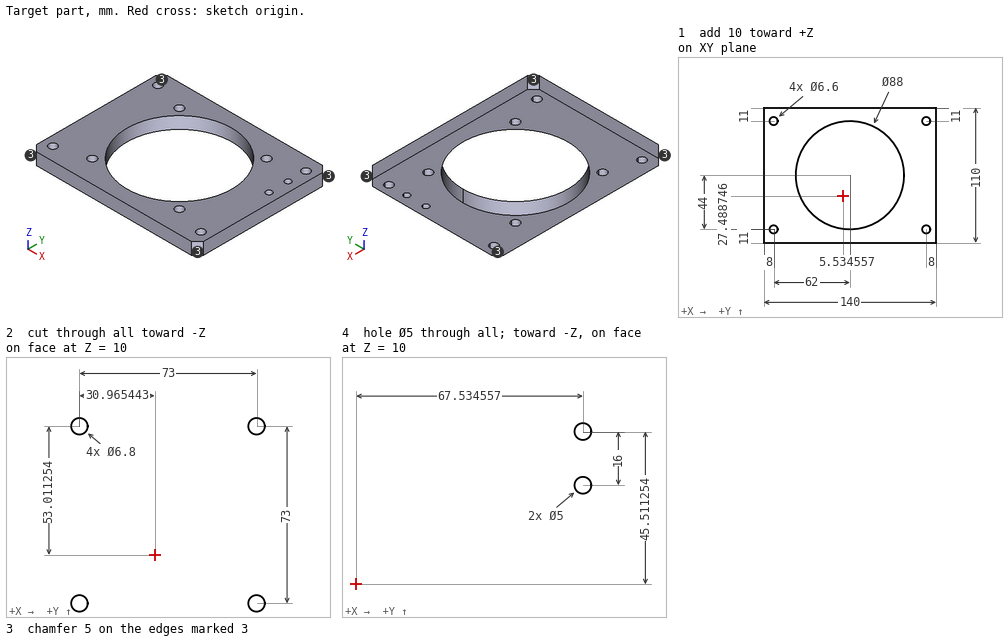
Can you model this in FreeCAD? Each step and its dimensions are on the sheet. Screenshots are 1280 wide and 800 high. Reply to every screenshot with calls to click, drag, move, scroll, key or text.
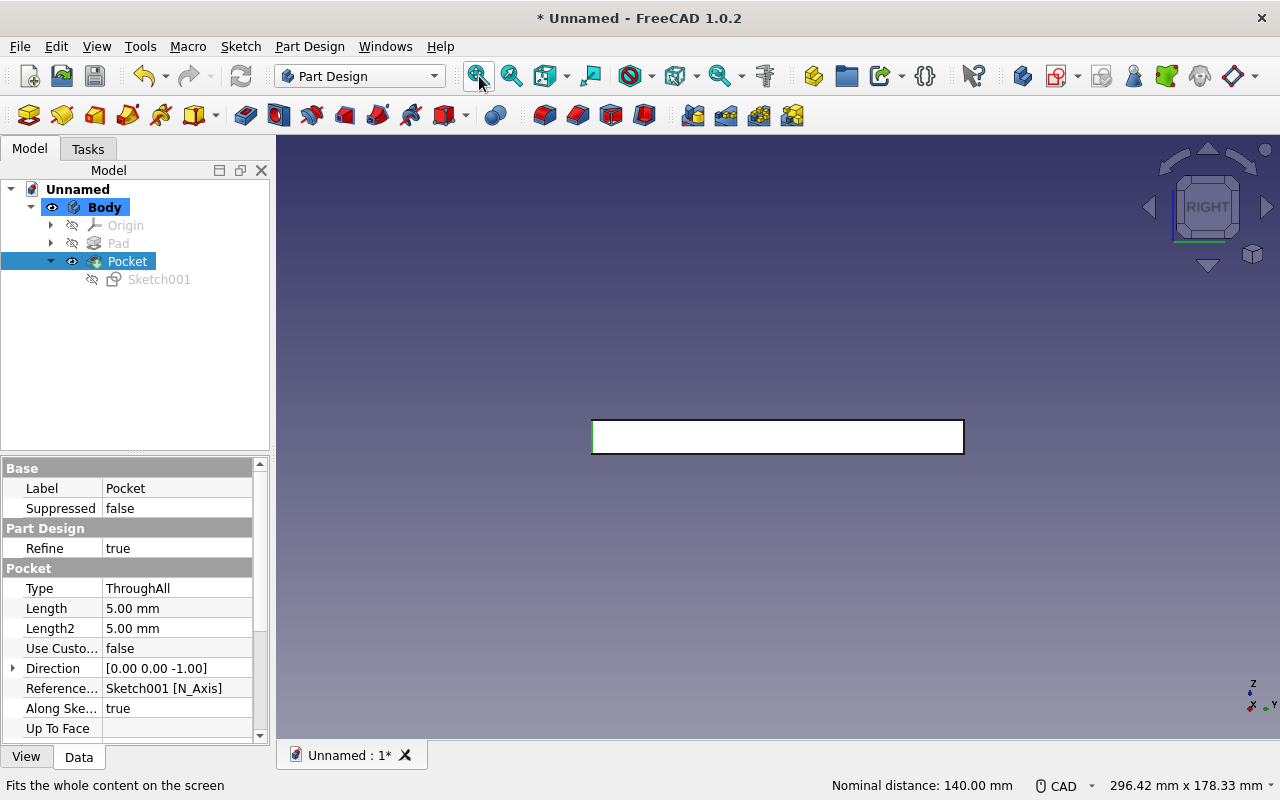
click(964, 436, ctrl)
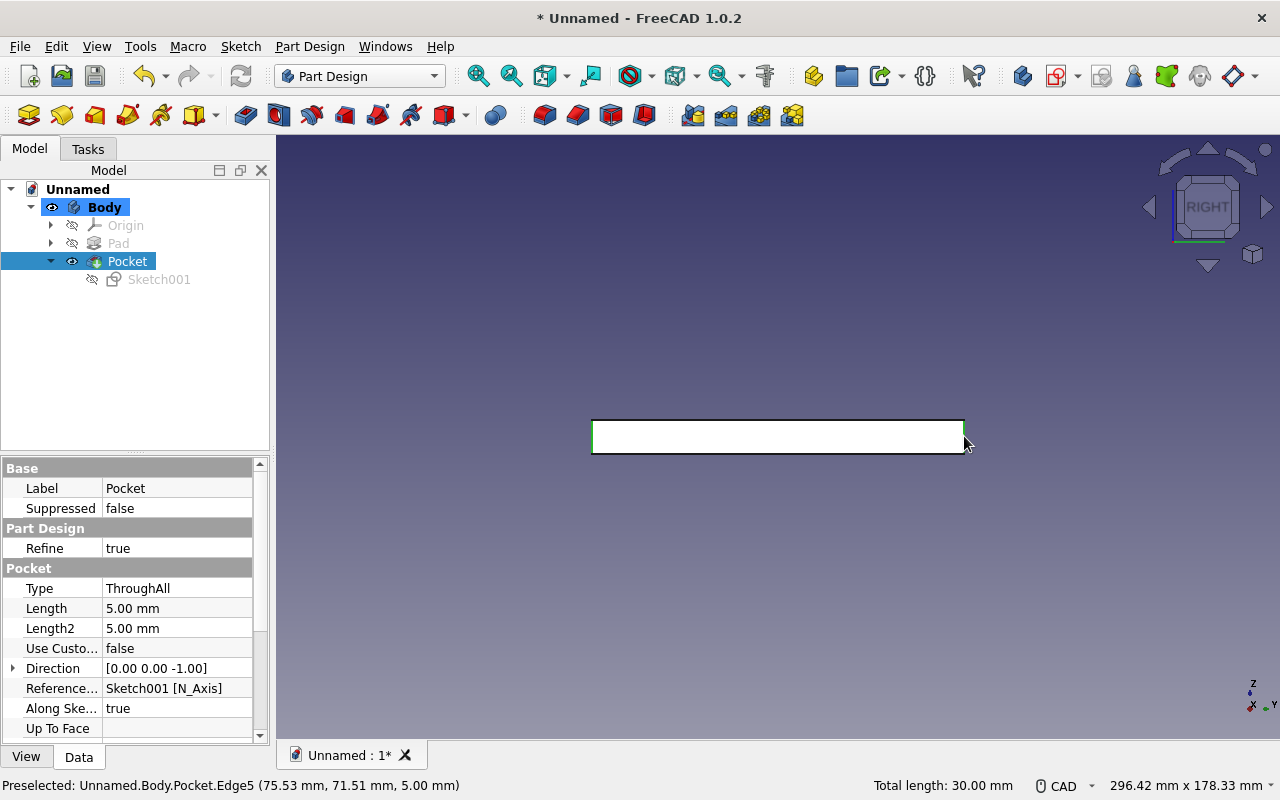
key(5)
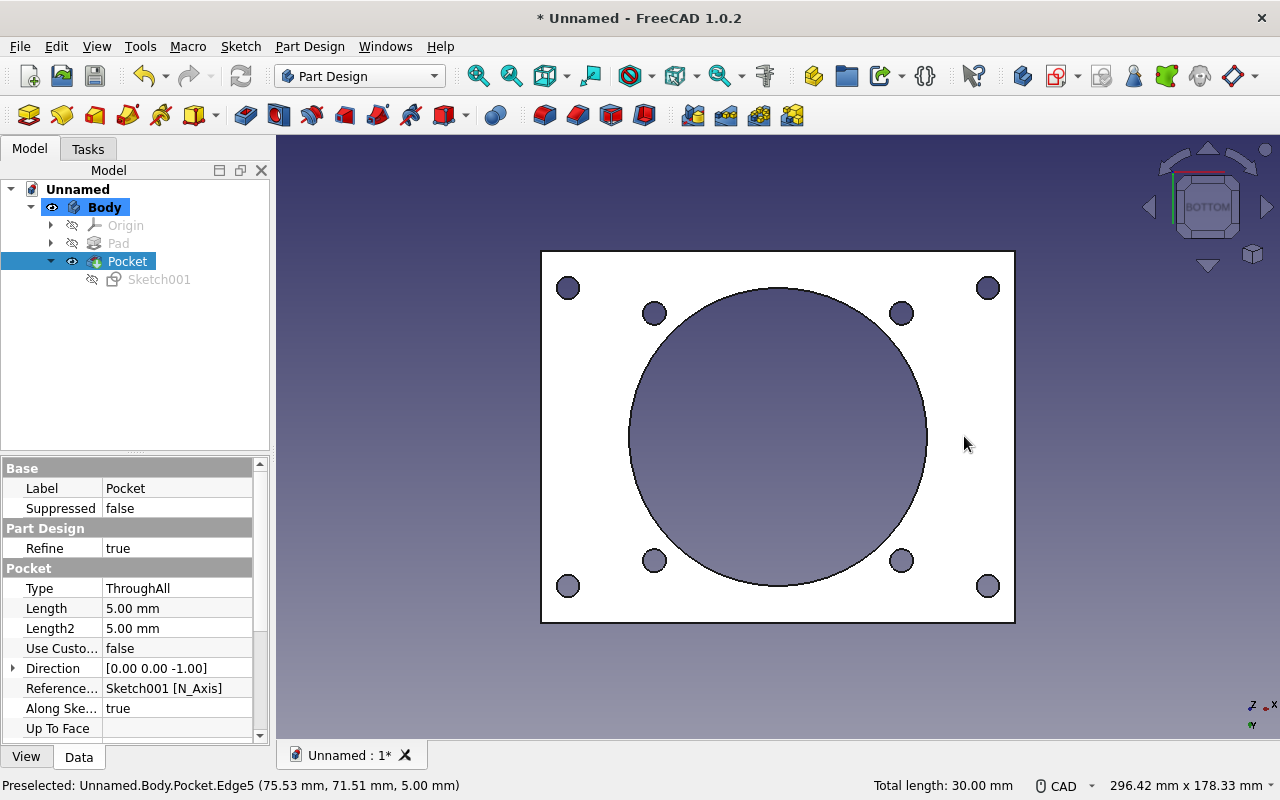
key(4)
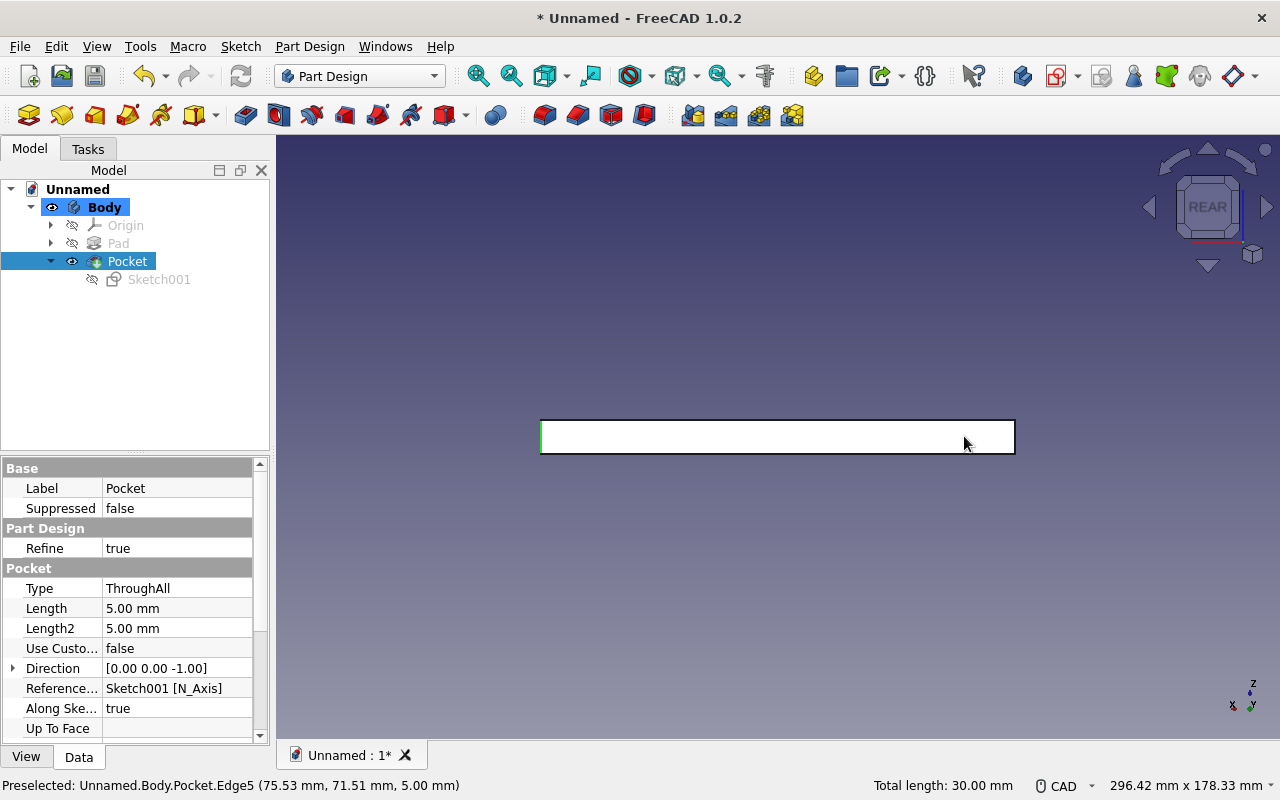
click(1015, 436, ctrl)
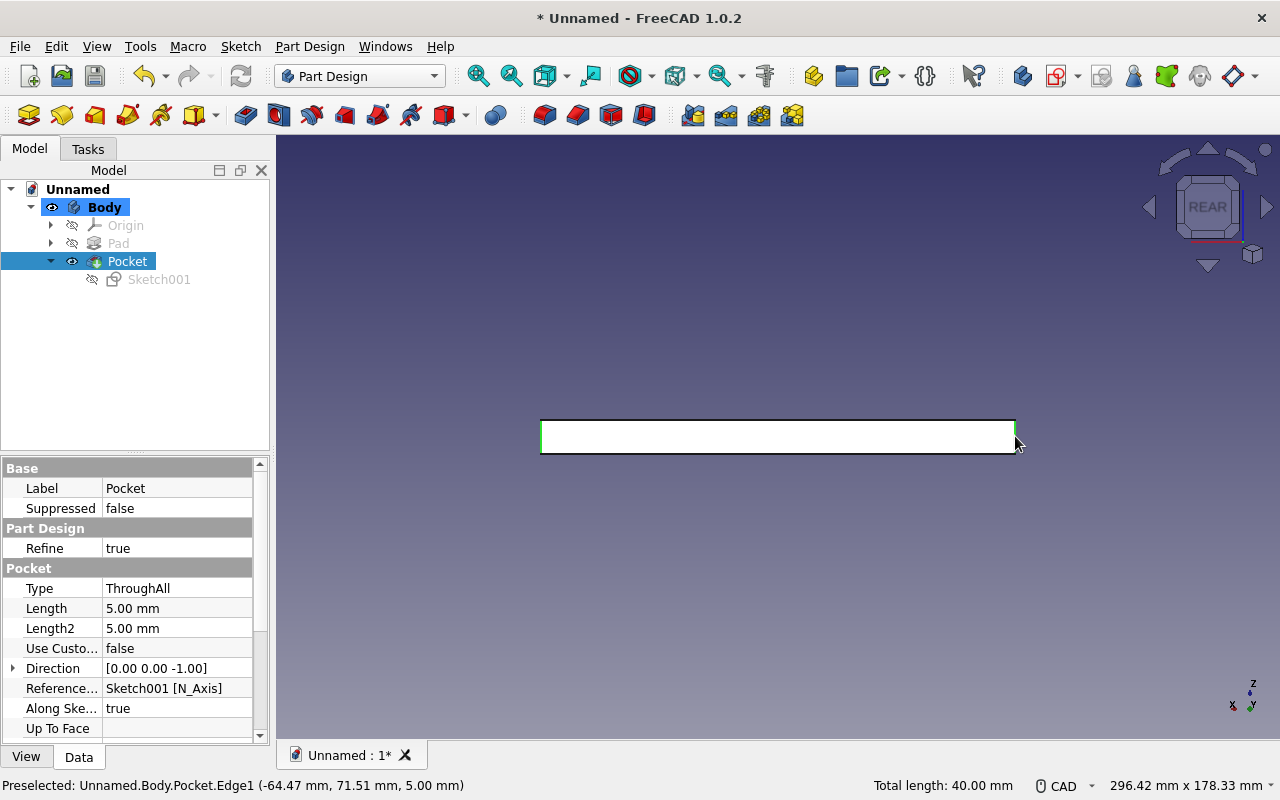
click(578, 116)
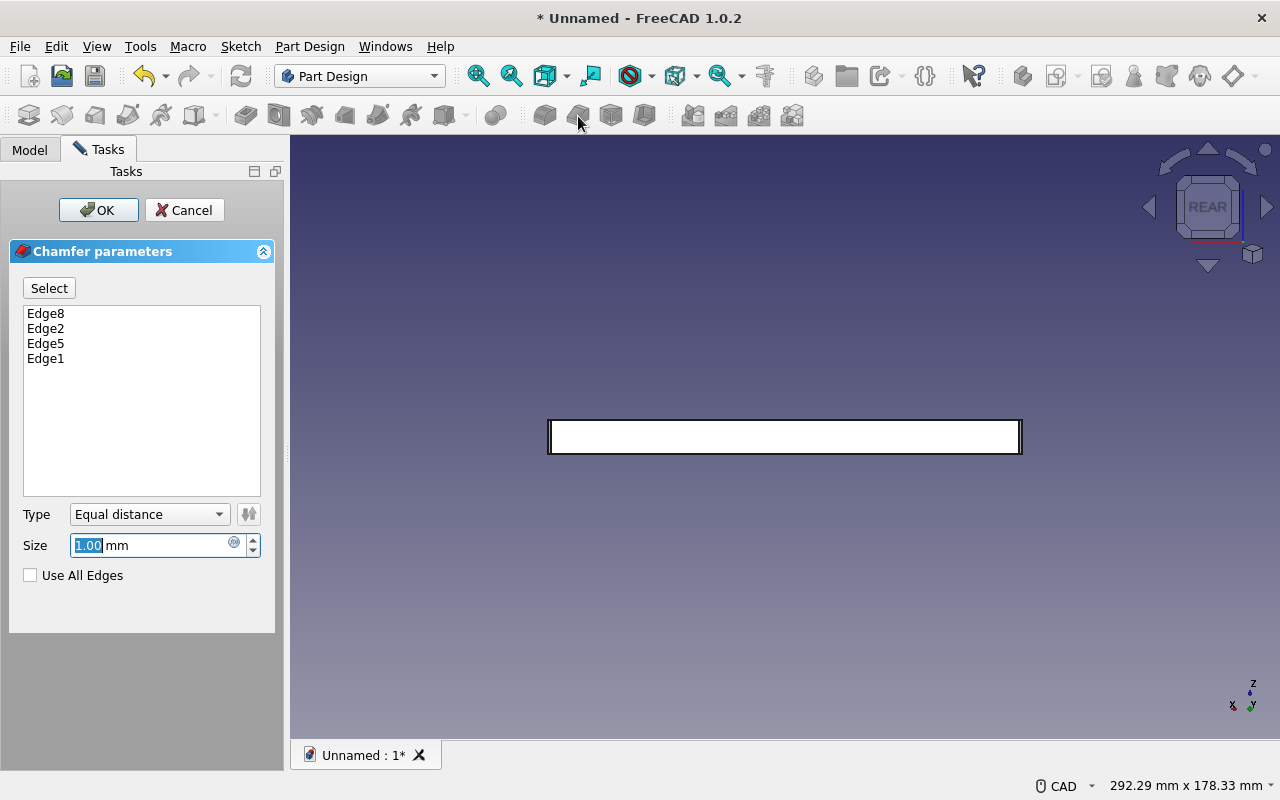
text(5)
key(Tab)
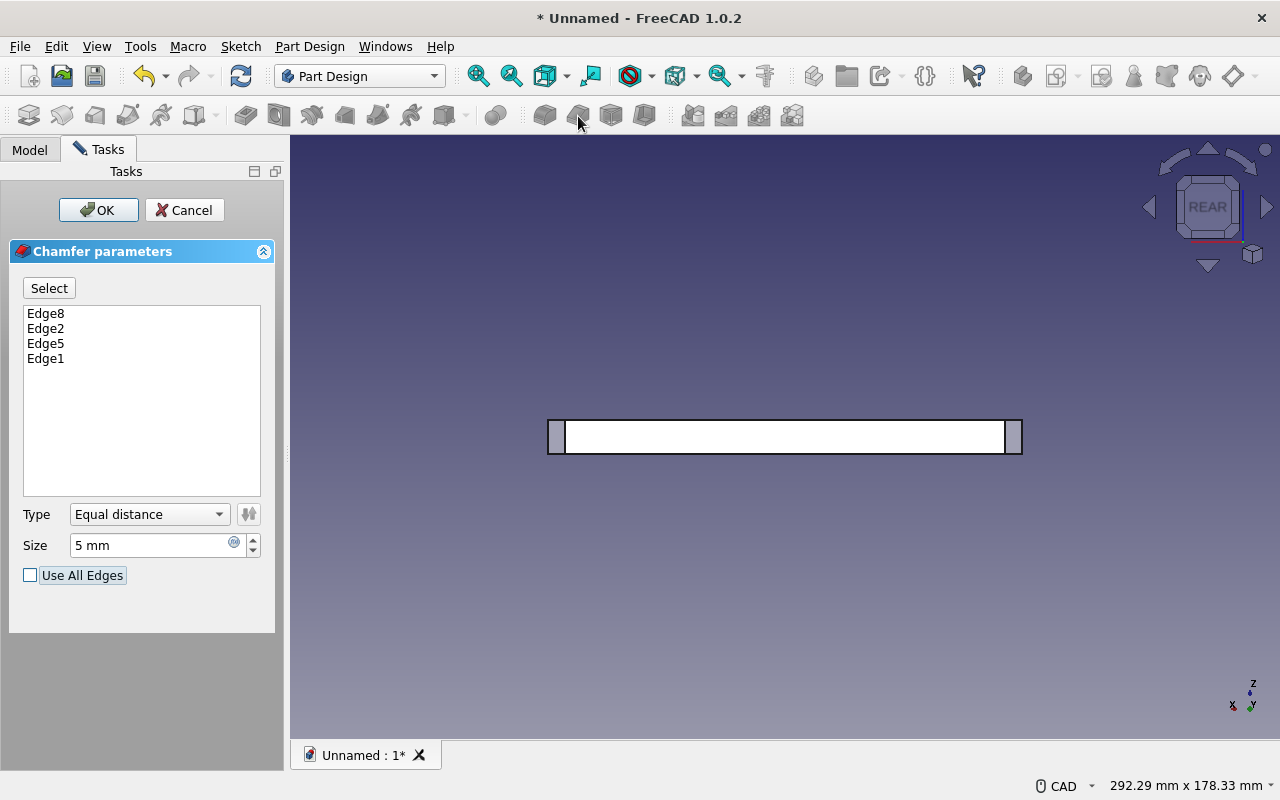
click(99, 210)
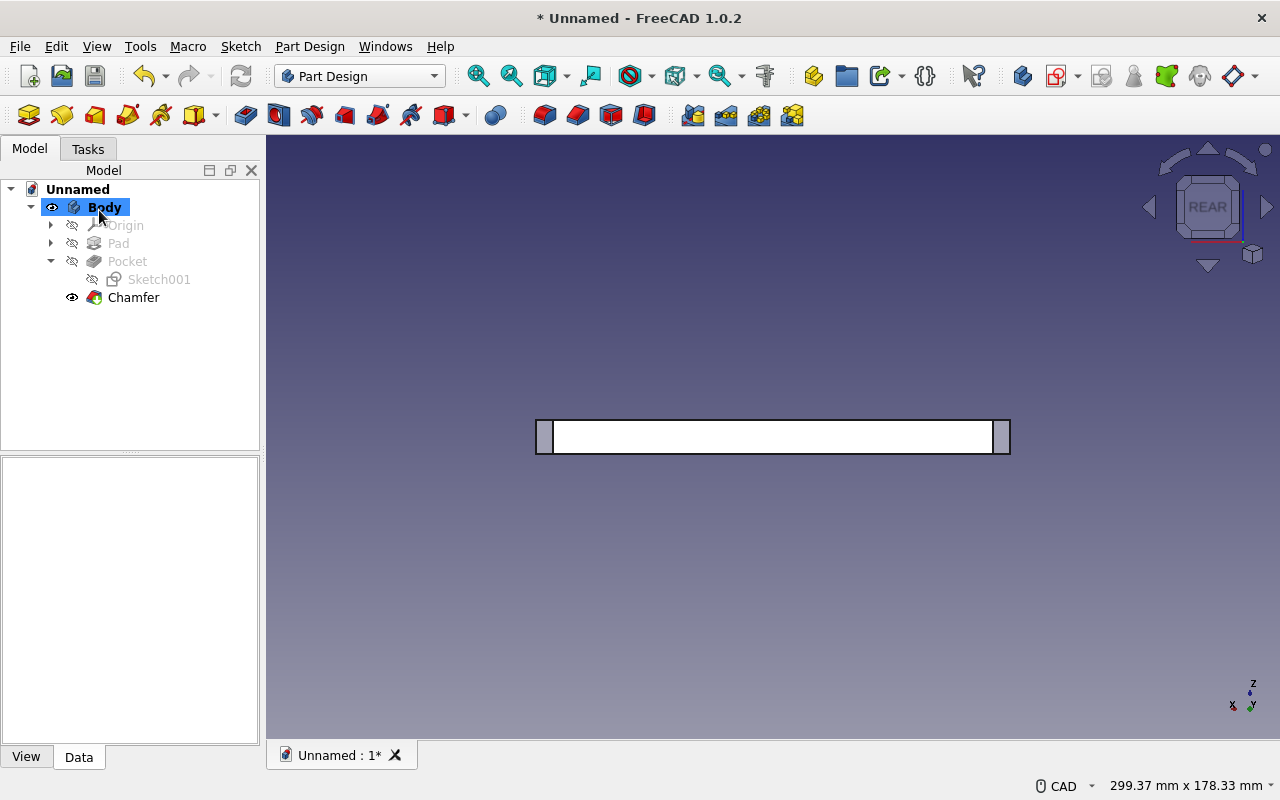
key(0)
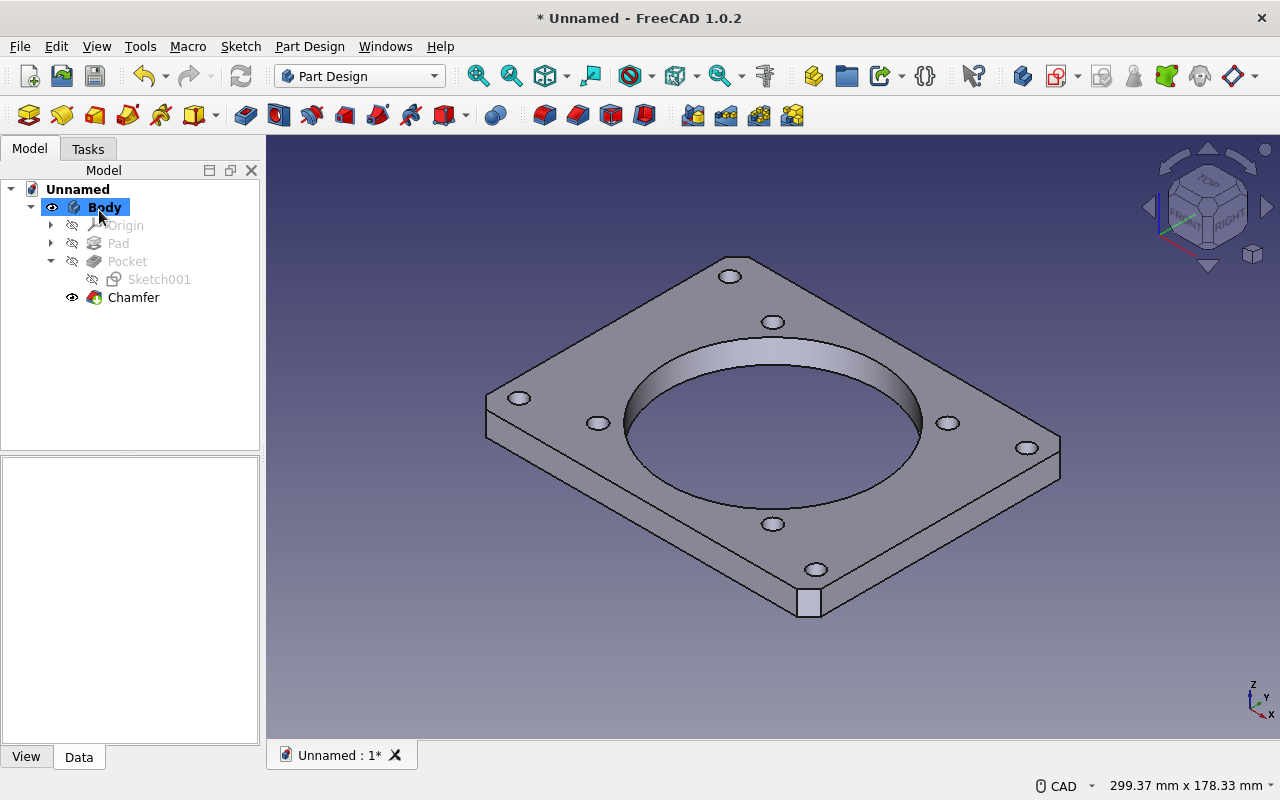
click(667, 317)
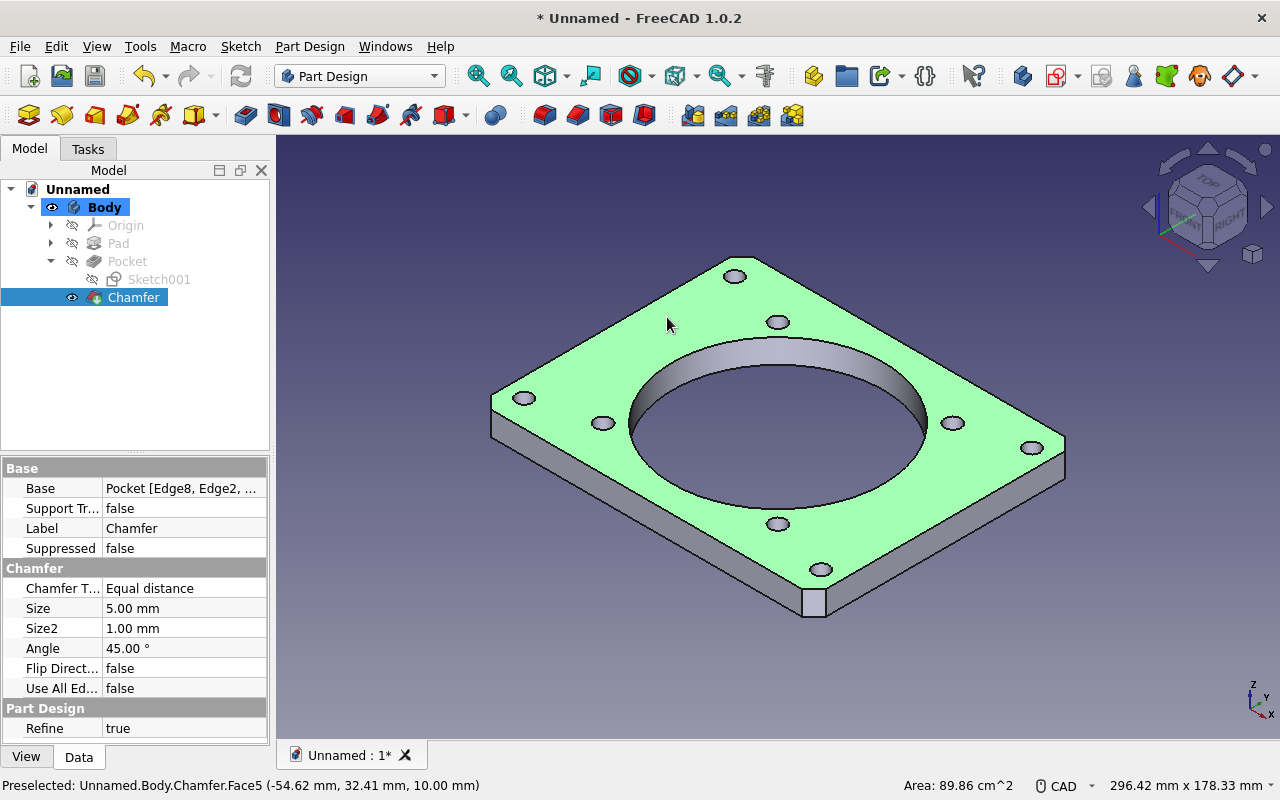
click(1056, 76)